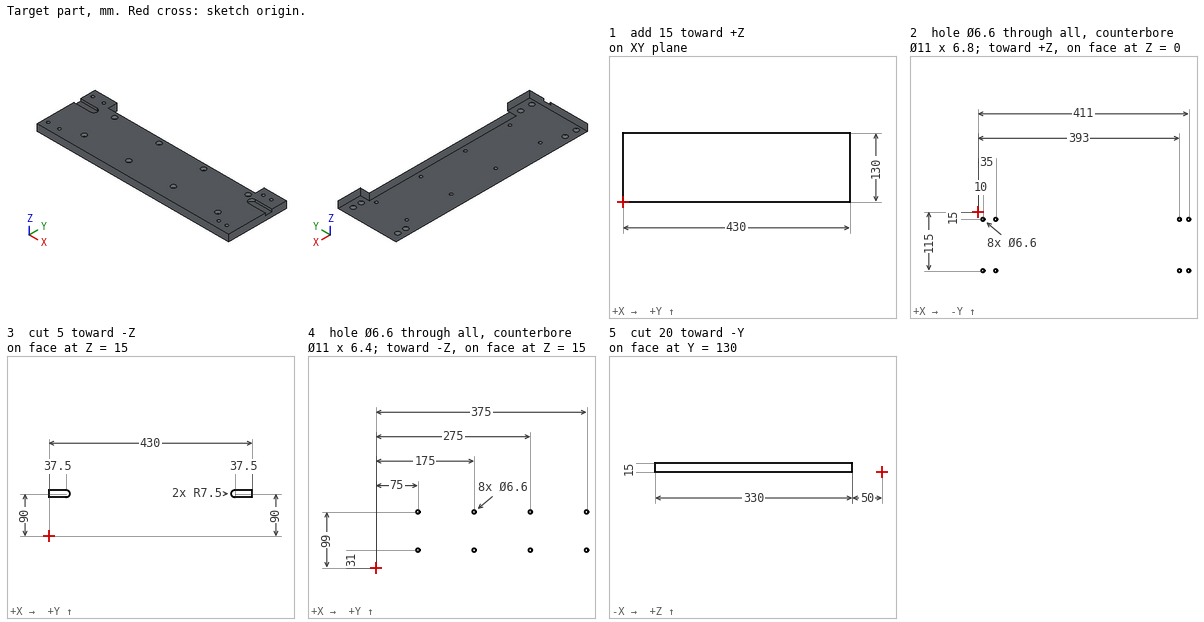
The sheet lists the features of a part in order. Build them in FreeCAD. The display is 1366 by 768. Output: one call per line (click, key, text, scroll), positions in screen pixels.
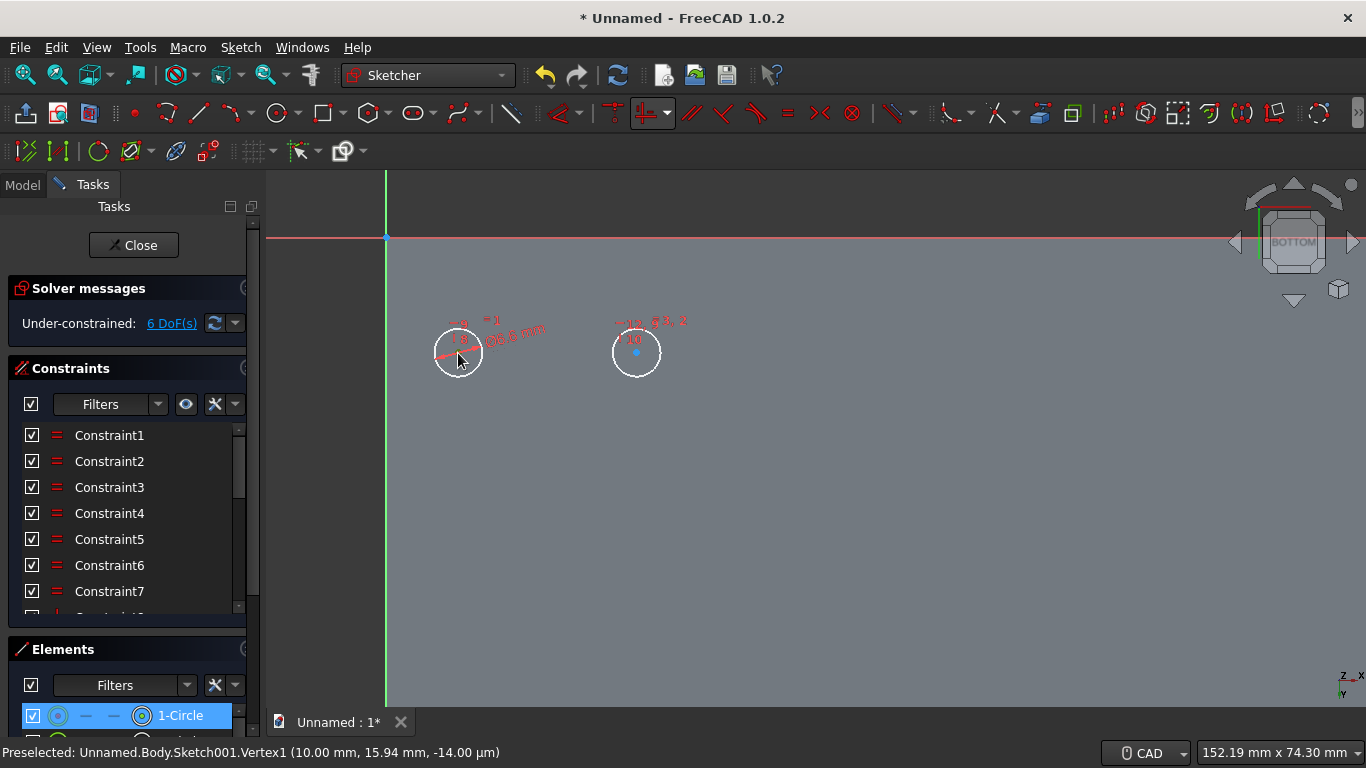
click(582, 114)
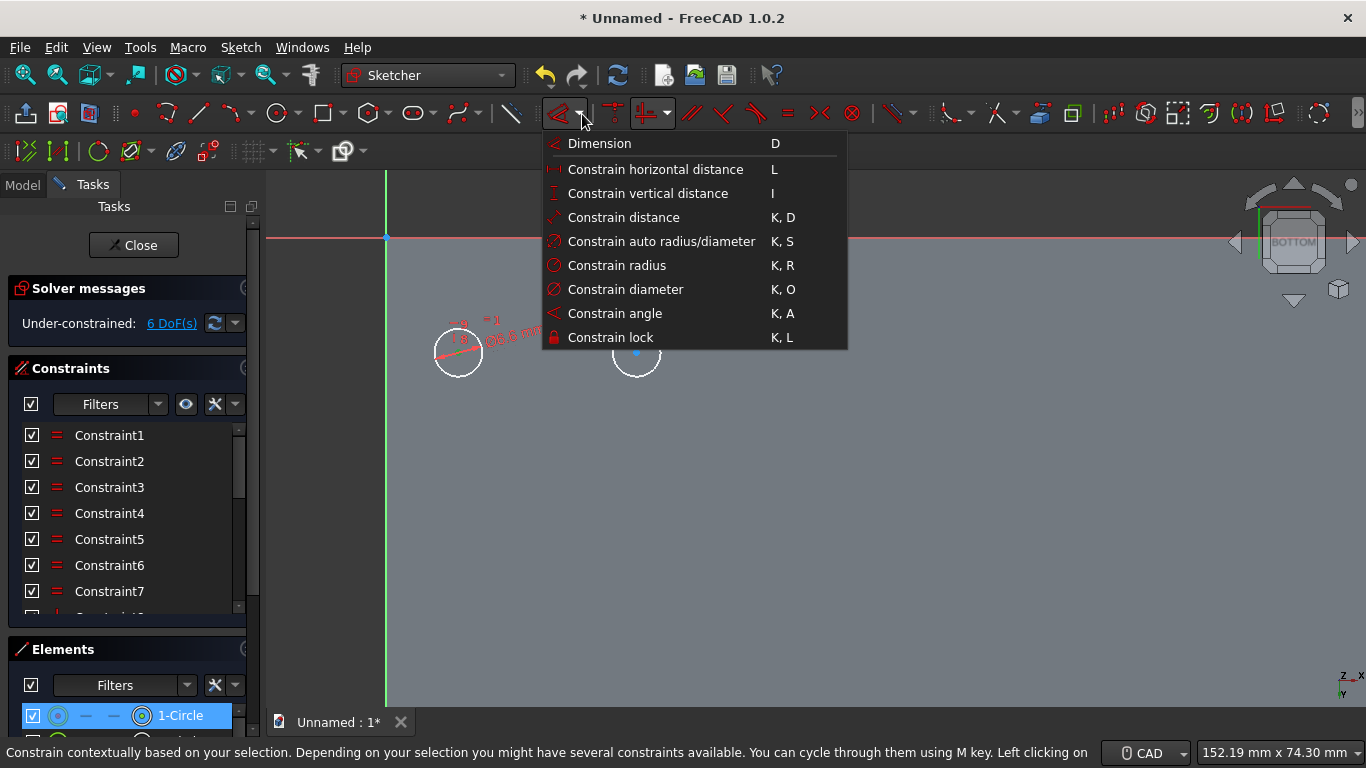
click(695, 169)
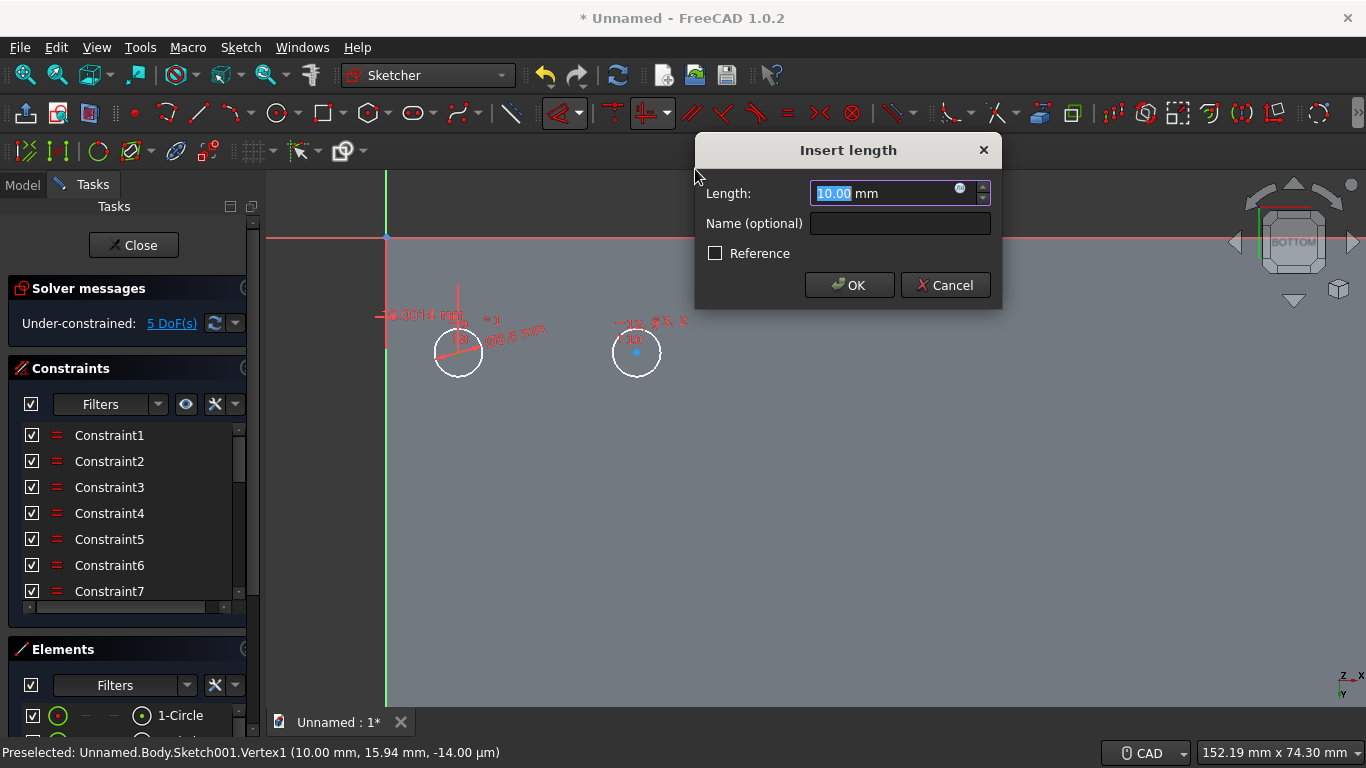
text(10)
key(Return)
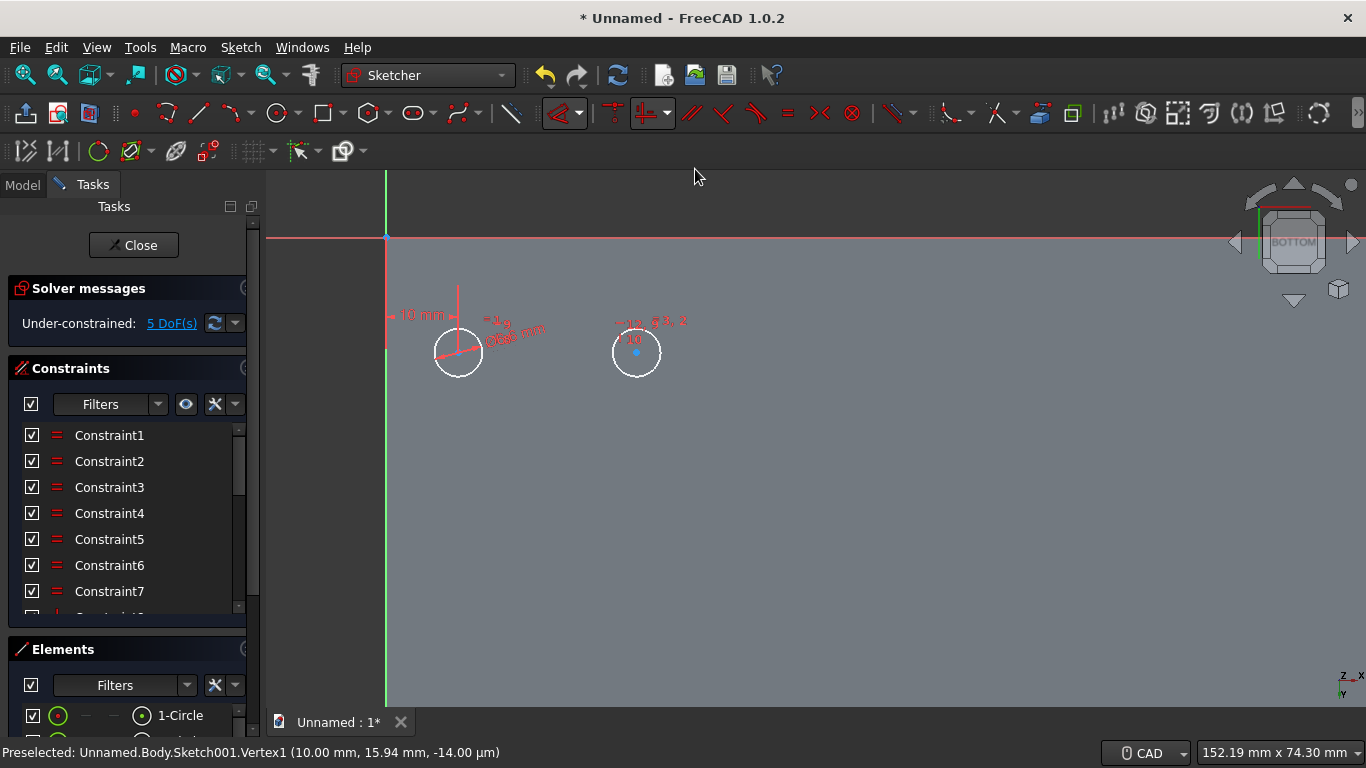
click(458, 353)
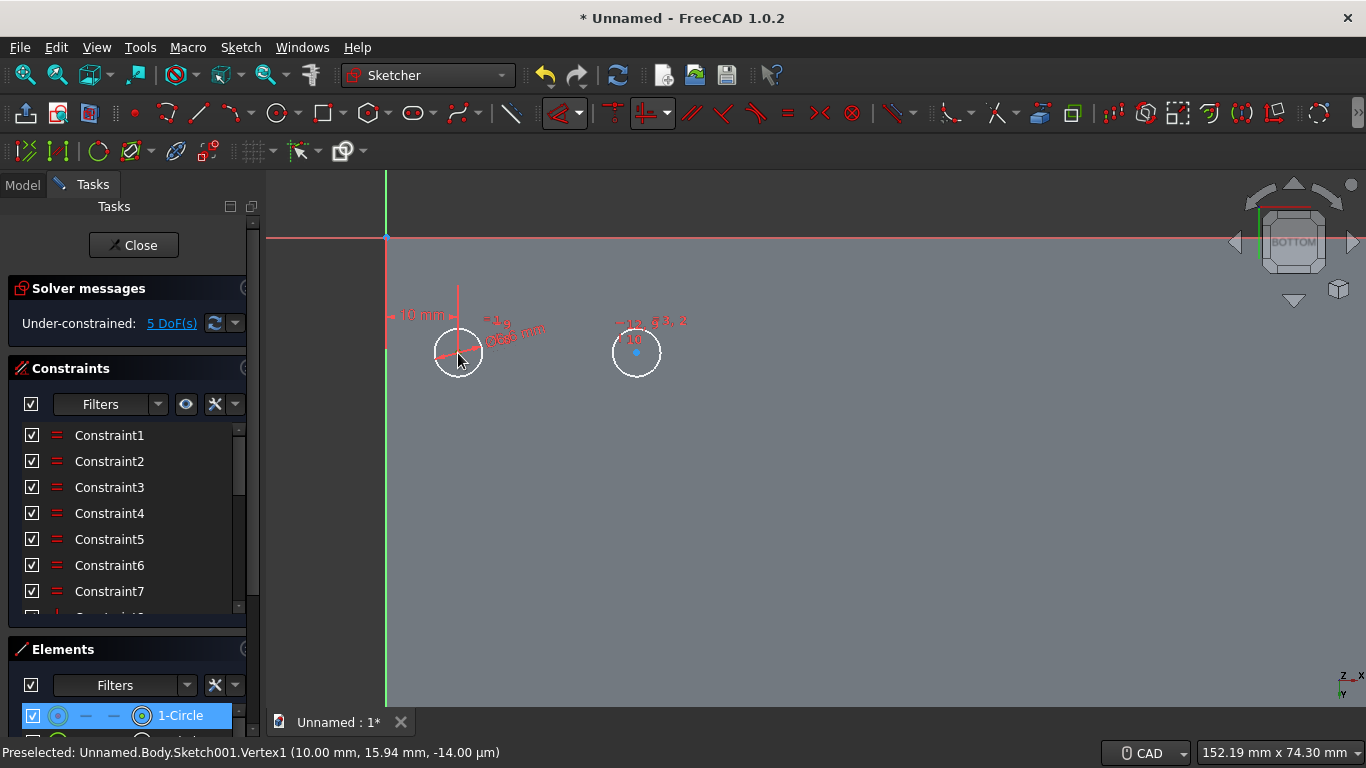
key(i)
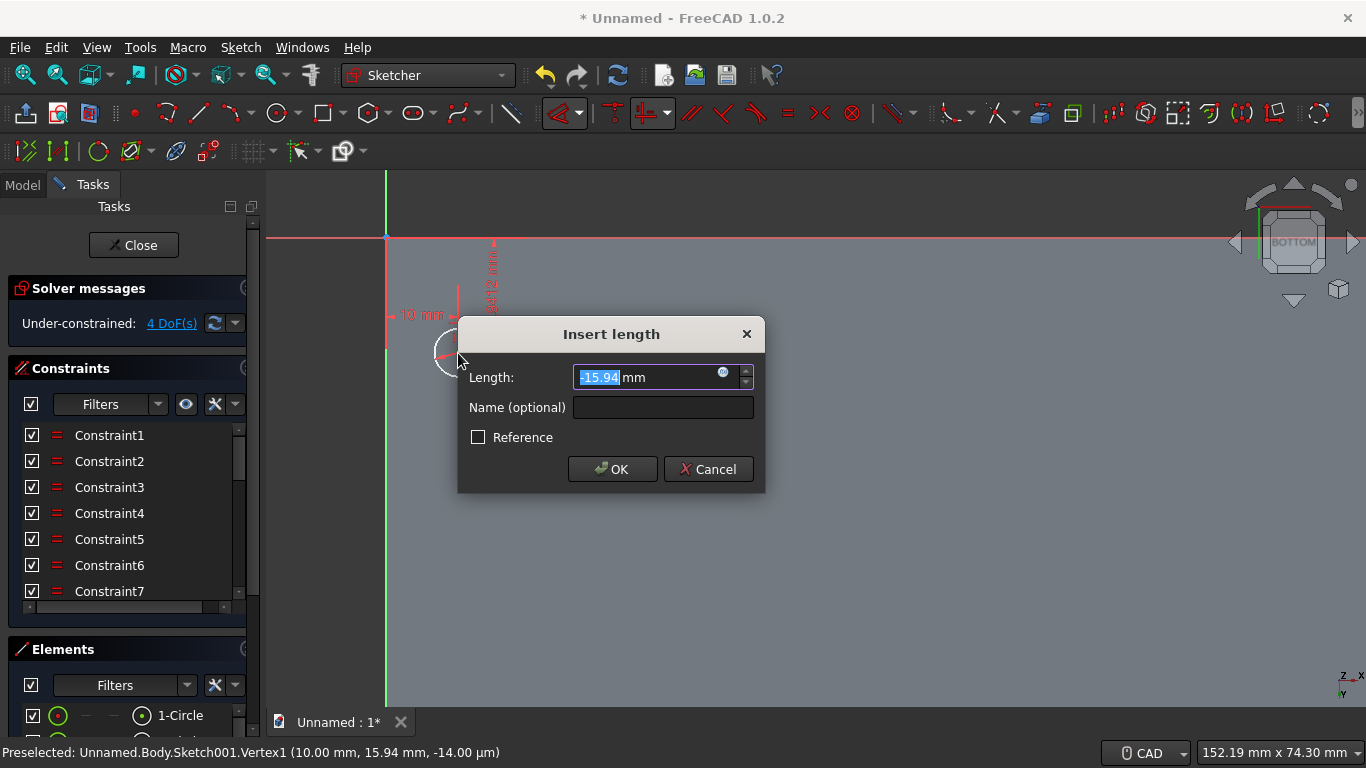
text(-15)
key(Return)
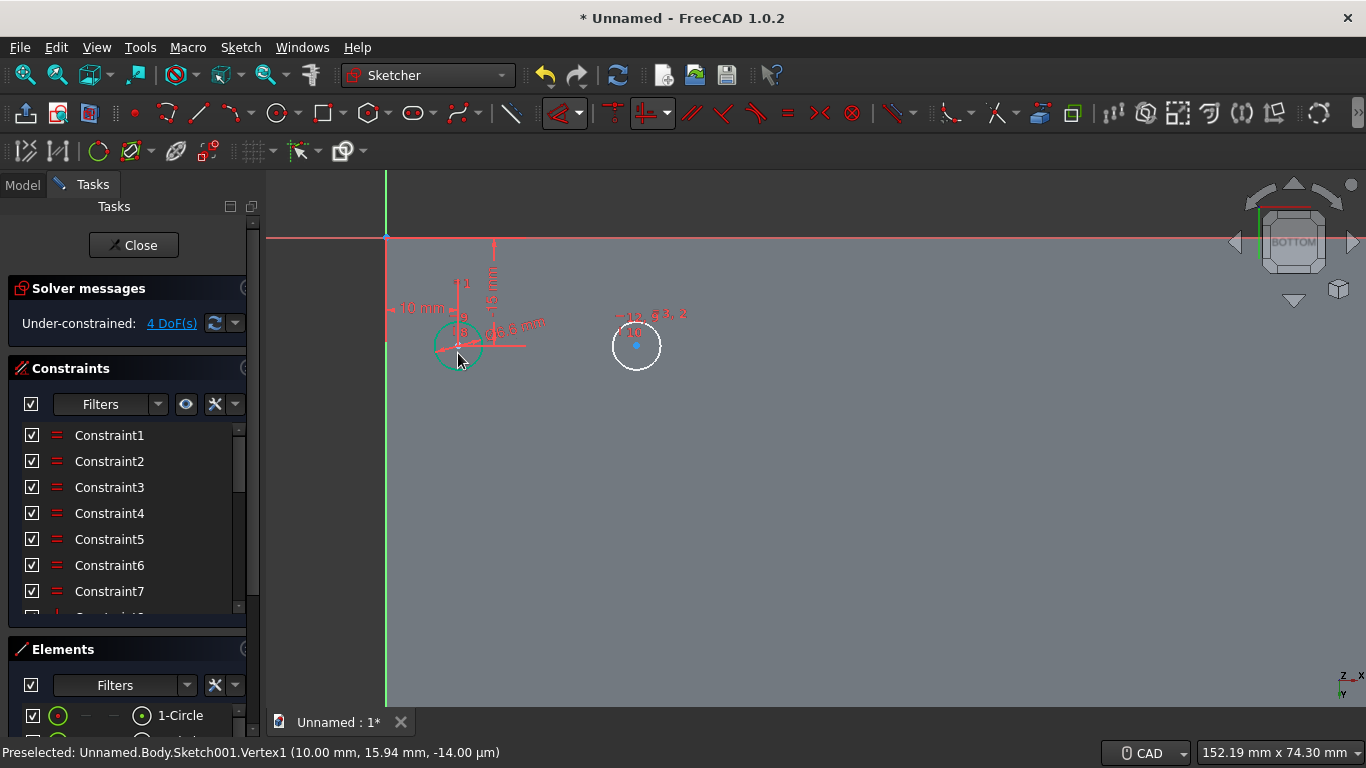
scroll(460, 381, down, 8)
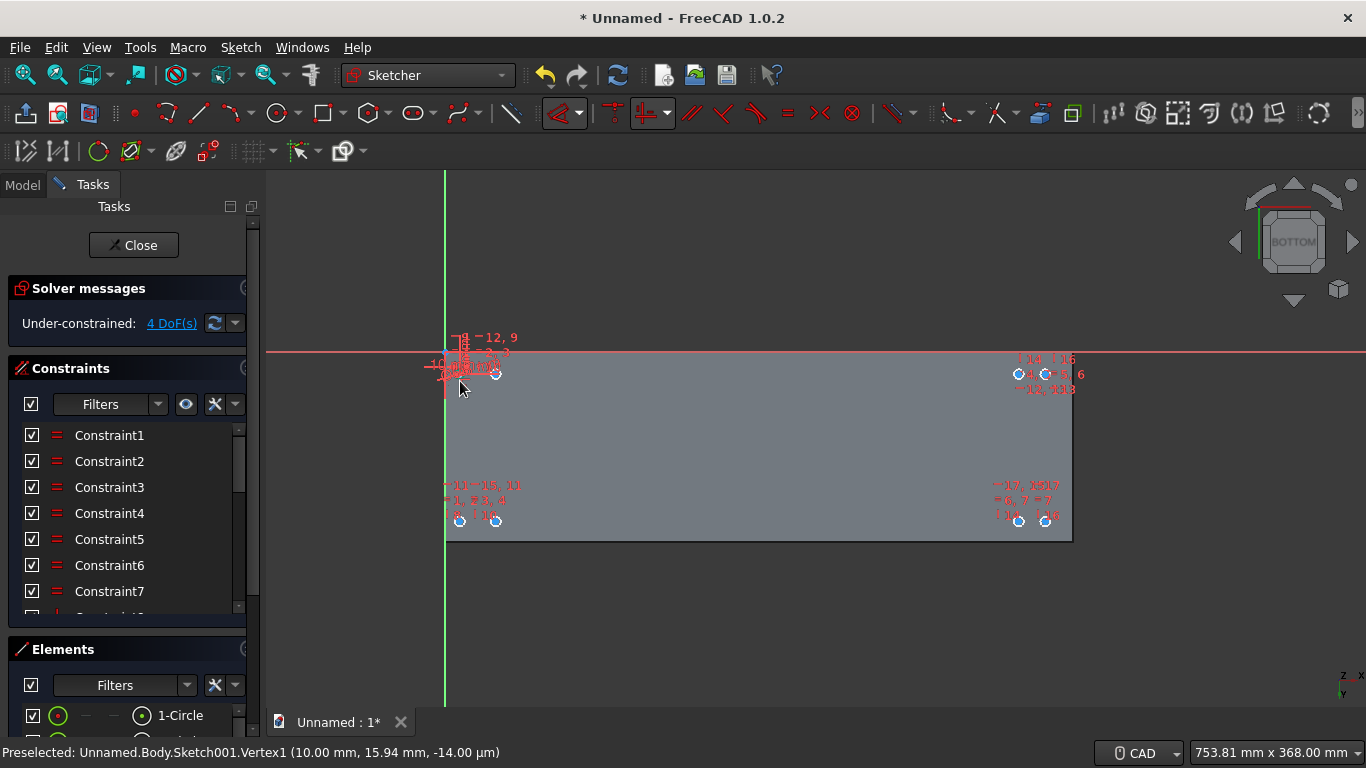
click(496, 374)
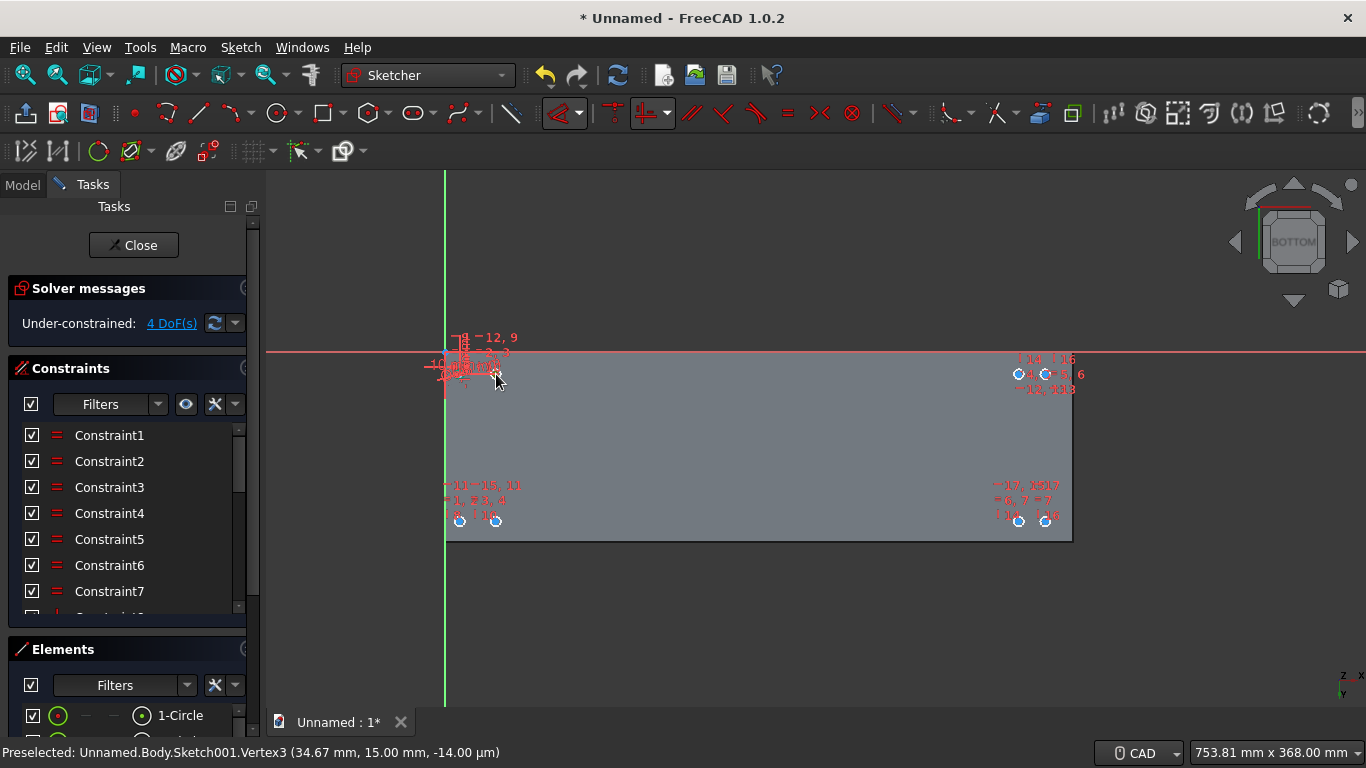
key(l)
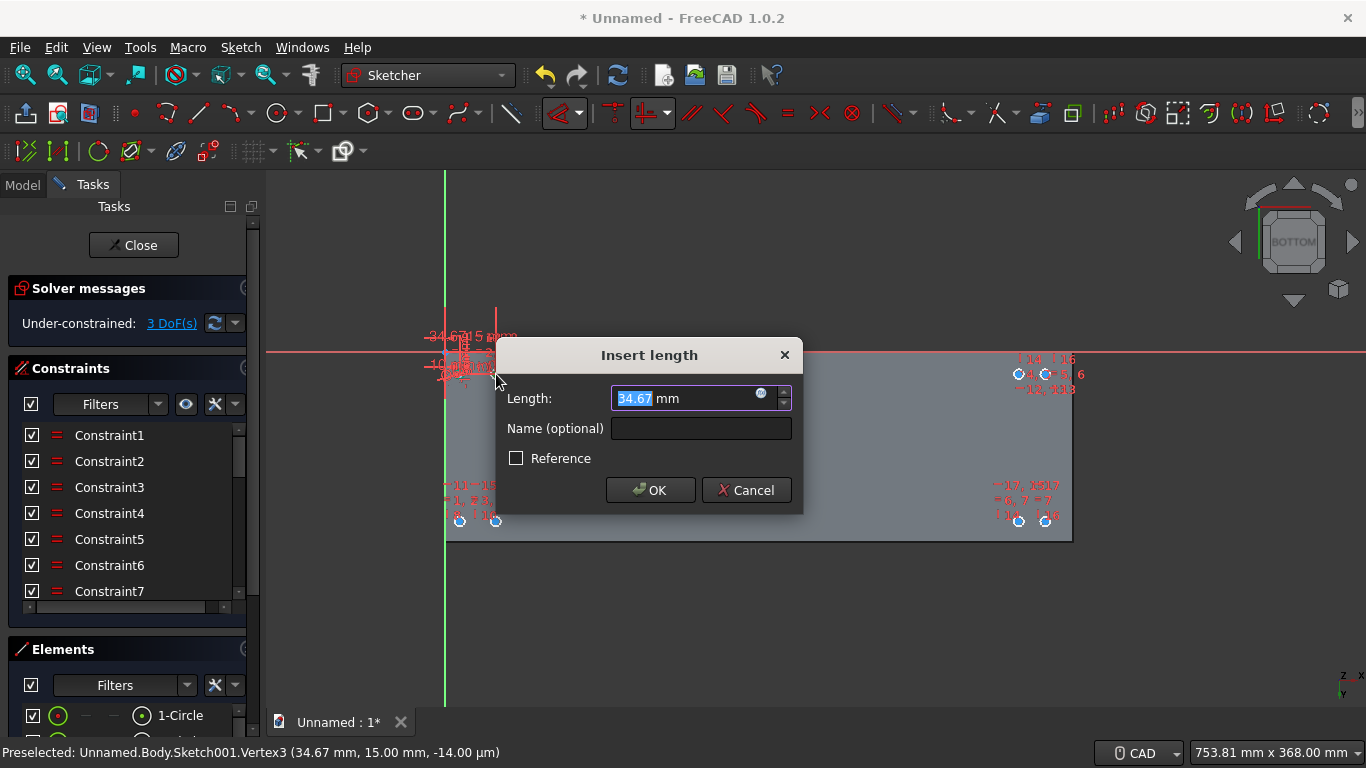
text(35)
key(Return)